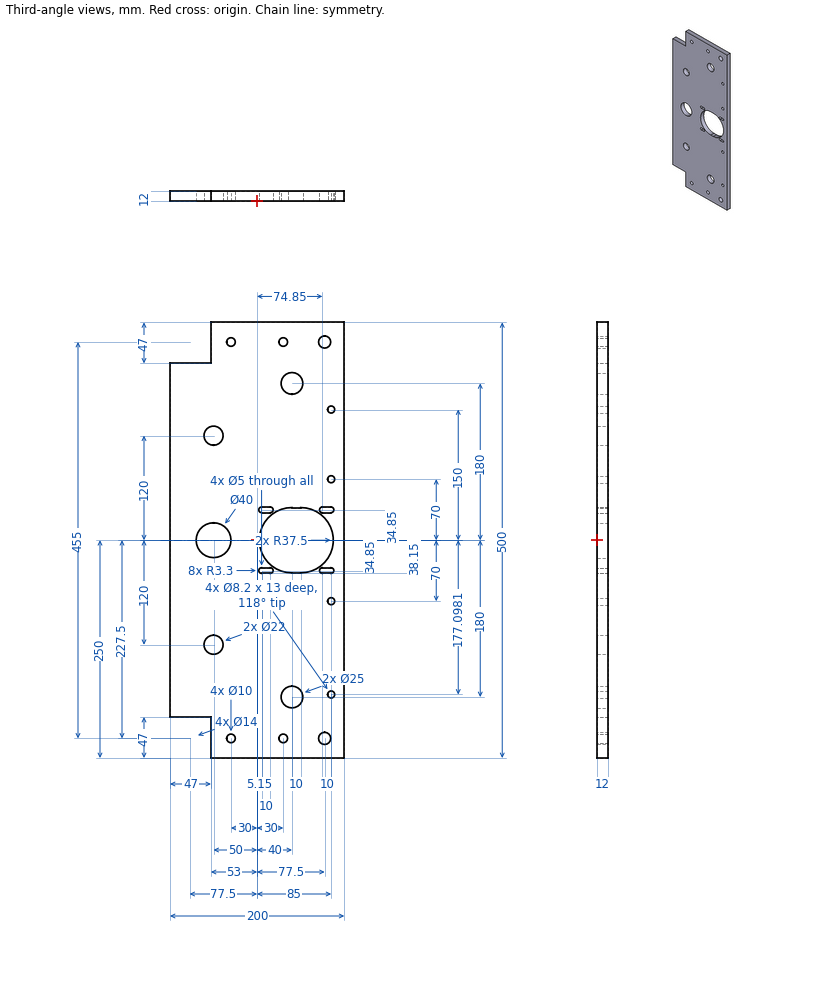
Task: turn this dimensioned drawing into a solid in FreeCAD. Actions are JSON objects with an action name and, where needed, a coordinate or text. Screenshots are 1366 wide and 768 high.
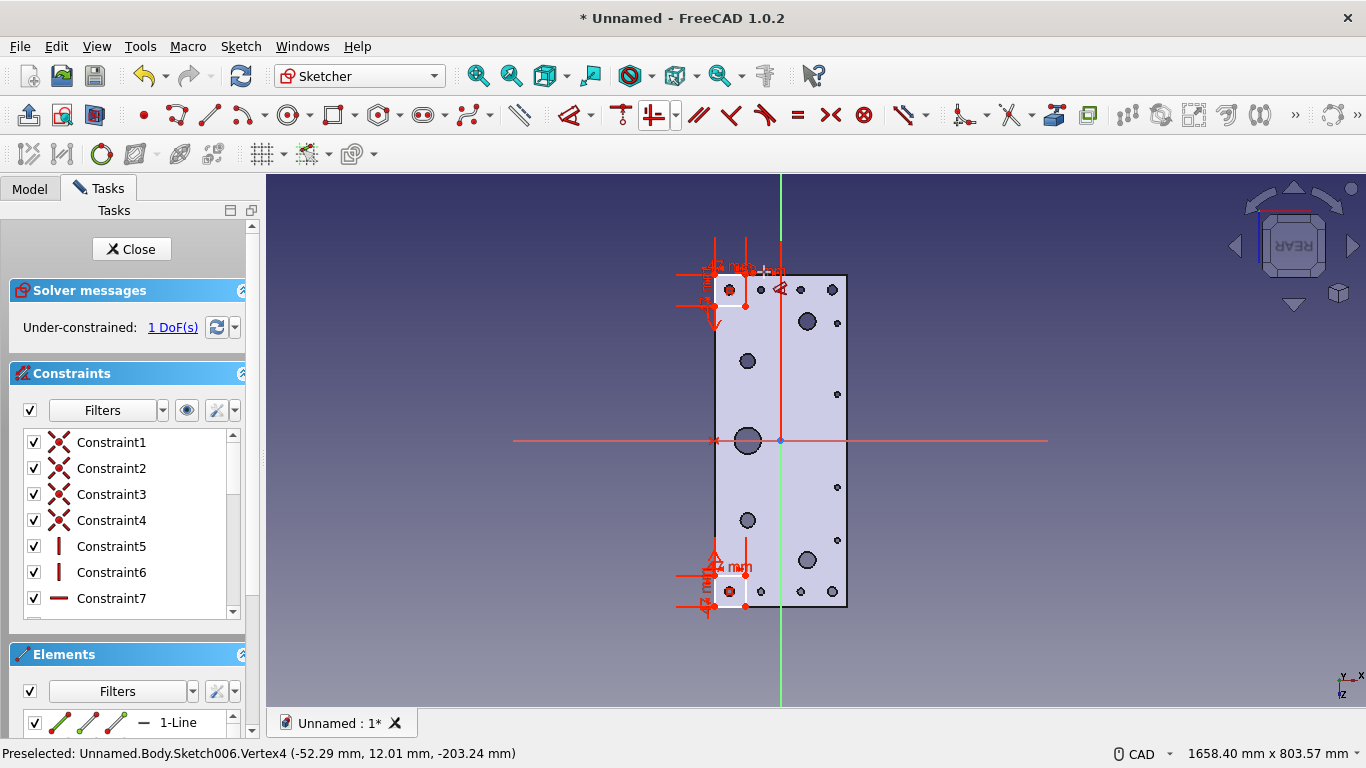
{"action": "left_click", "coordinate": [715, 275]}
{"action": "left_click", "coordinate": [815, 358]}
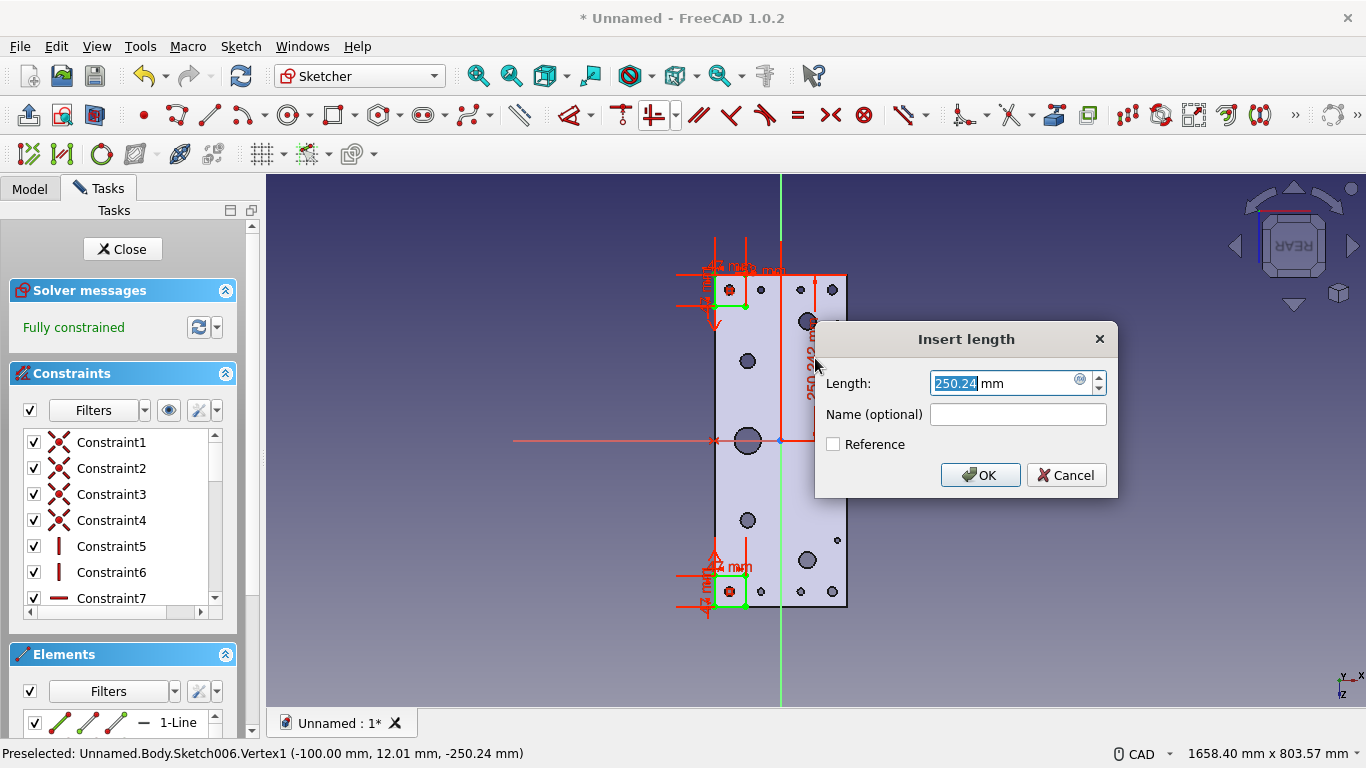
{"action": "type", "text": "250"}
{"action": "key", "text": "Return"}
{"action": "key", "text": "Escape"}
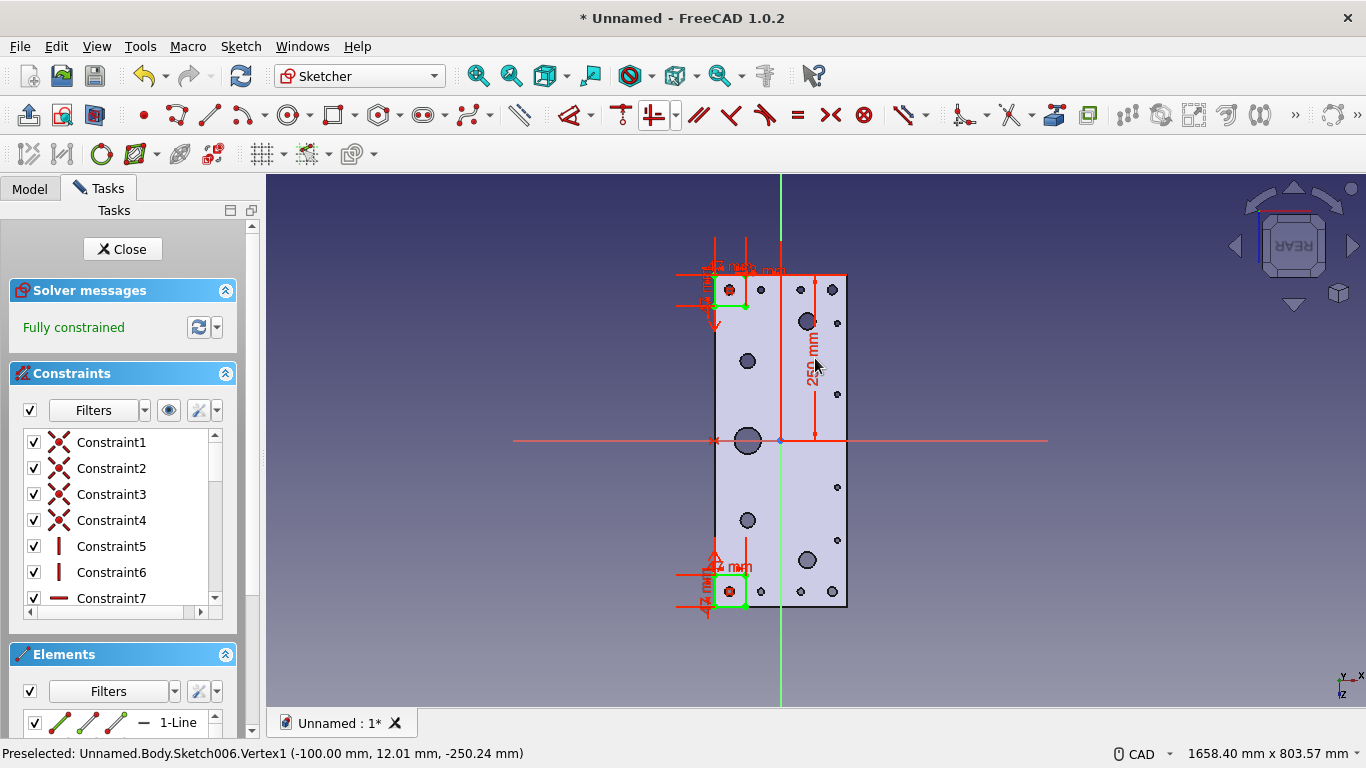
{"action": "left_click", "coordinate": [123, 249]}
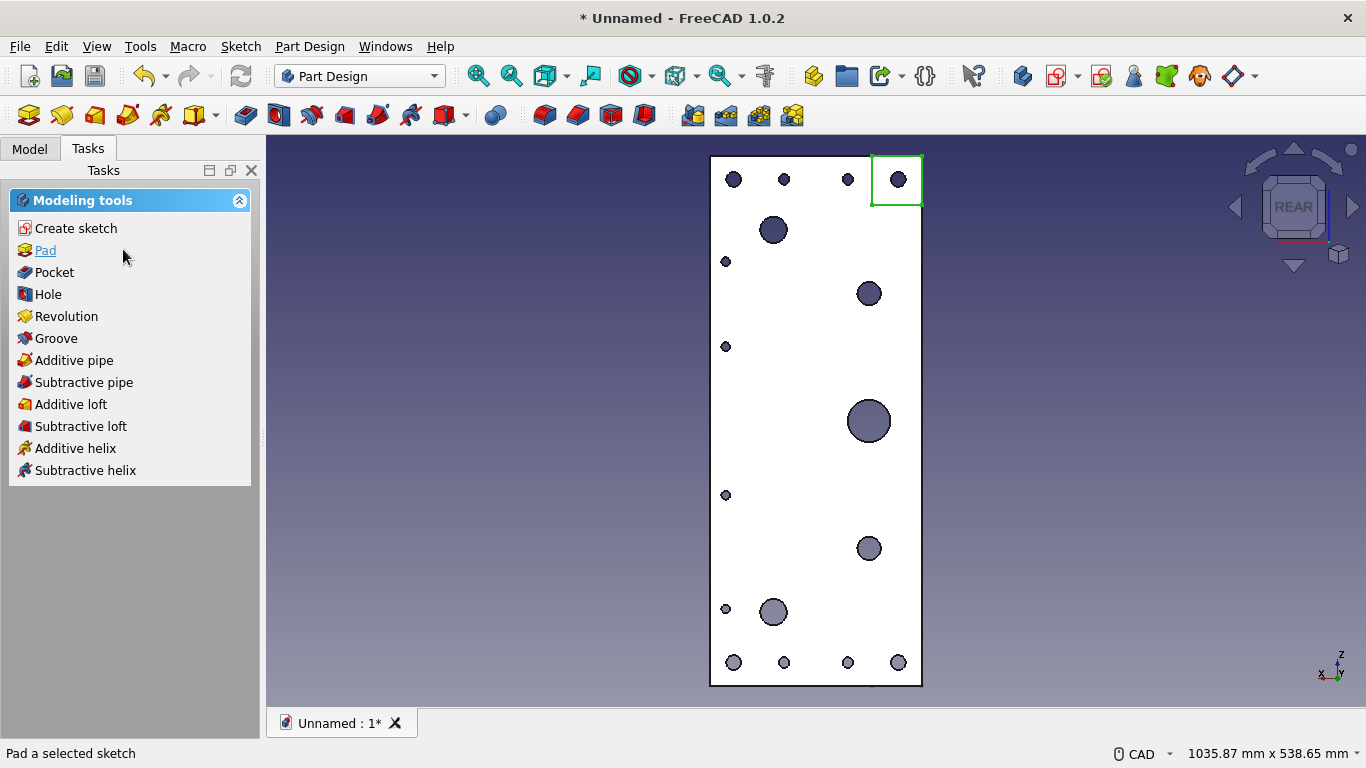
{"action": "left_click", "coordinate": [246, 116]}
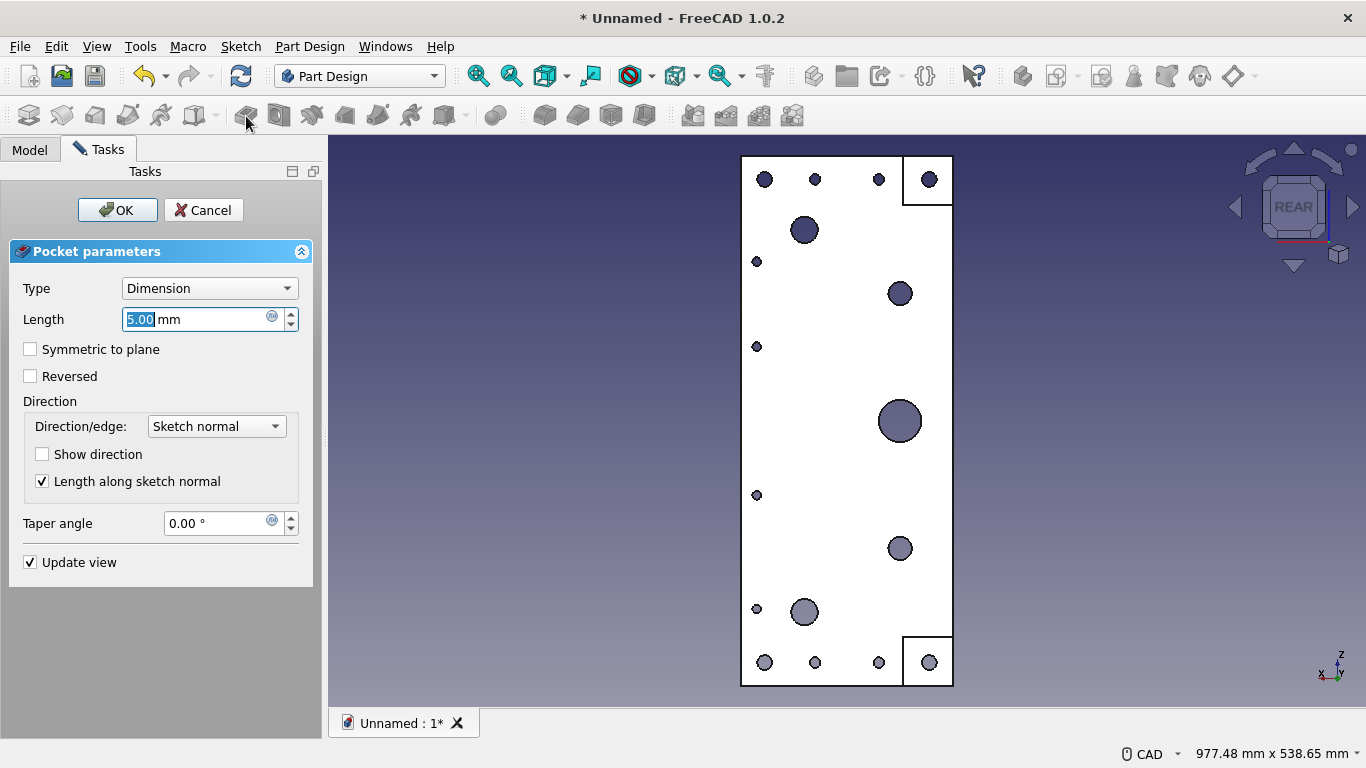
{"action": "left_click", "coordinate": [210, 288]}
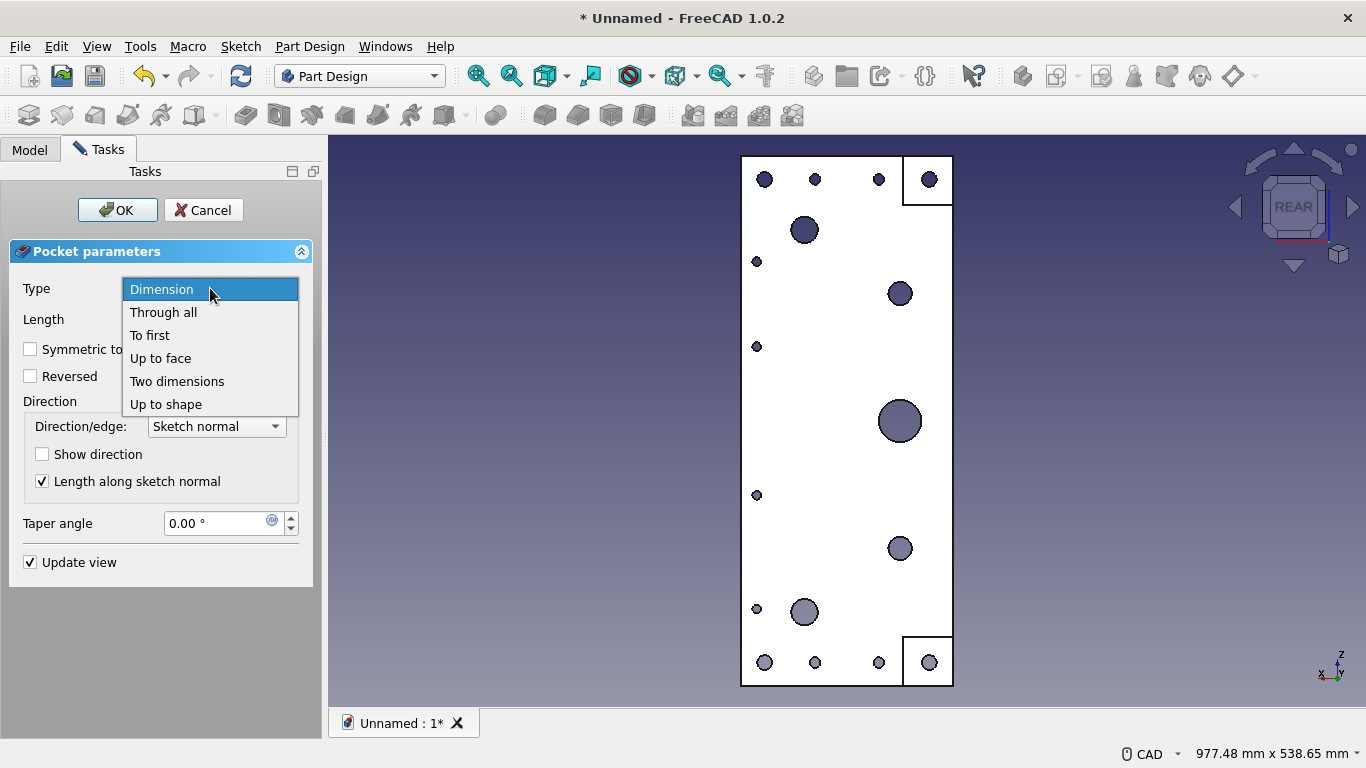
{"action": "left_click", "coordinate": [208, 312]}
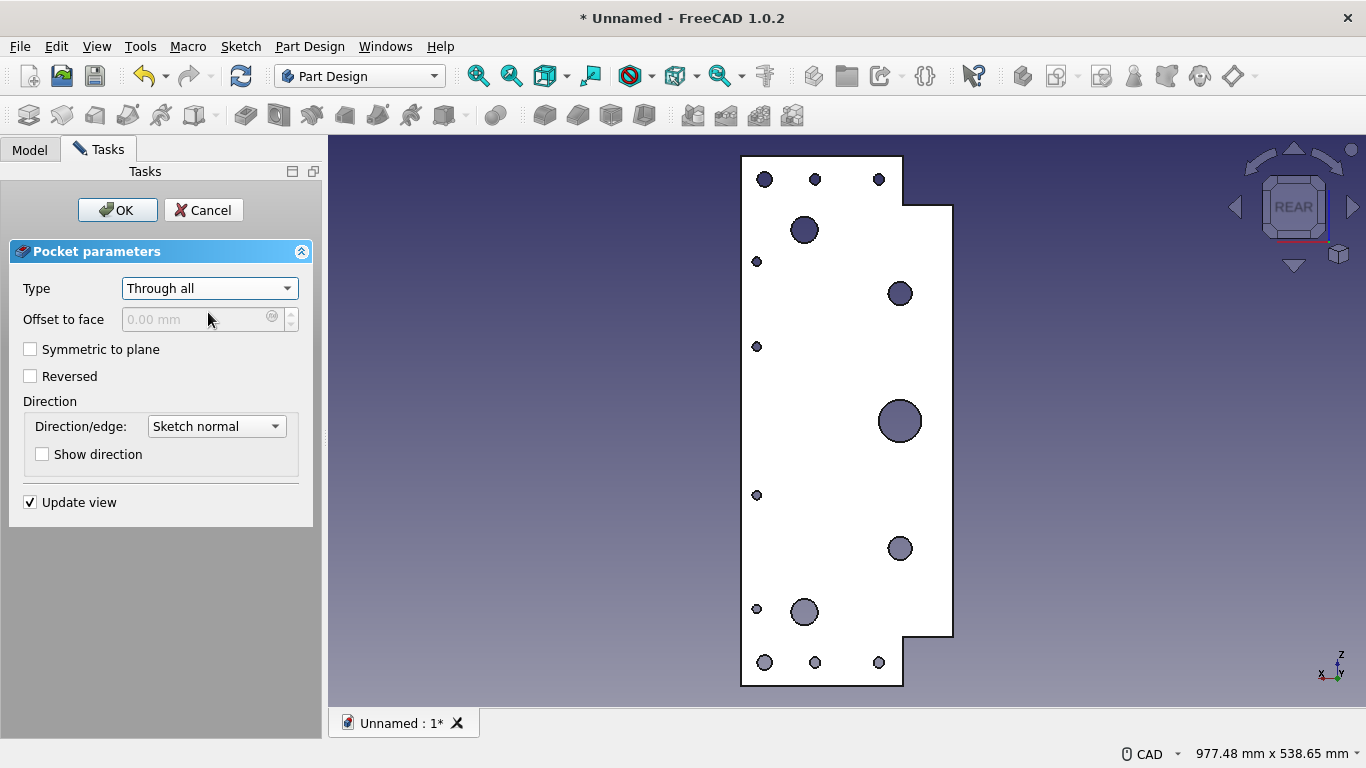
{"action": "left_click", "coordinate": [118, 210]}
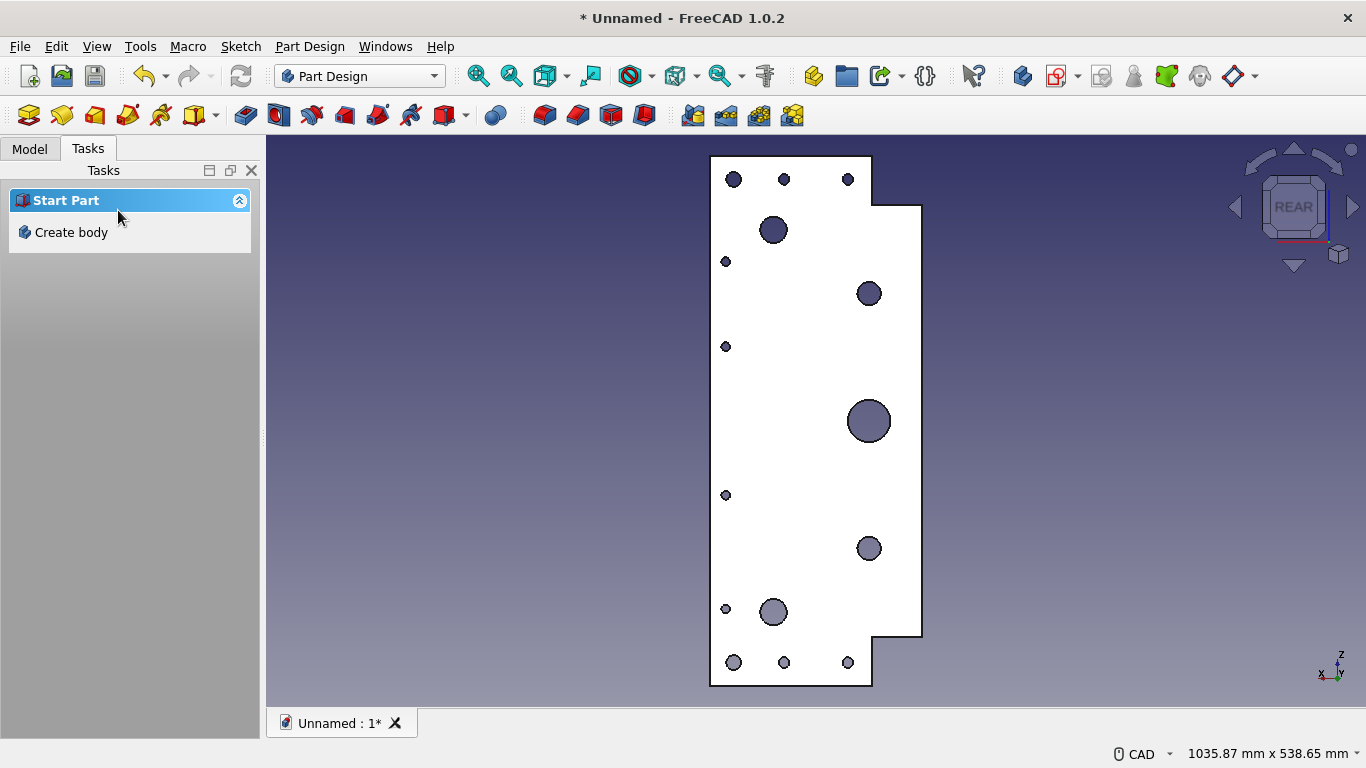
{"action": "left_click", "coordinate": [816, 496]}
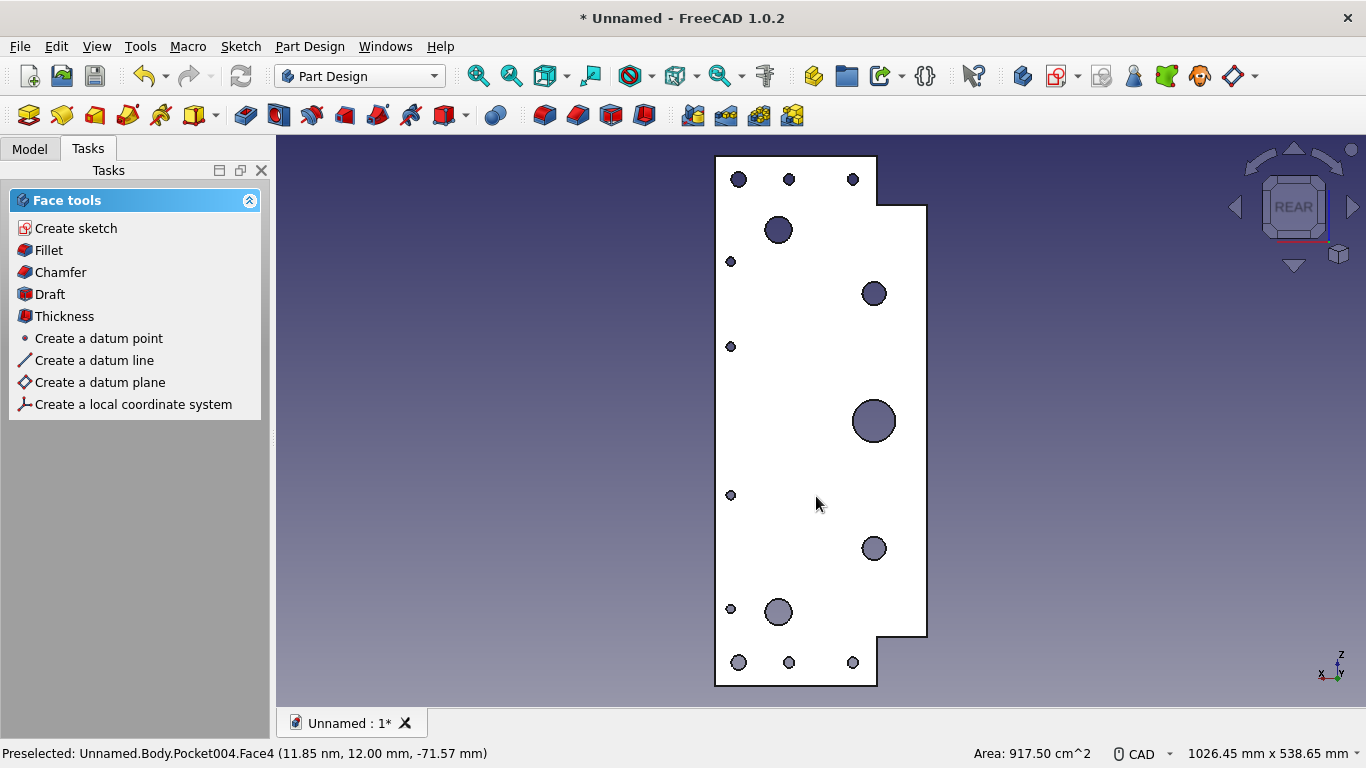
{"action": "left_click", "coordinate": [1056, 76]}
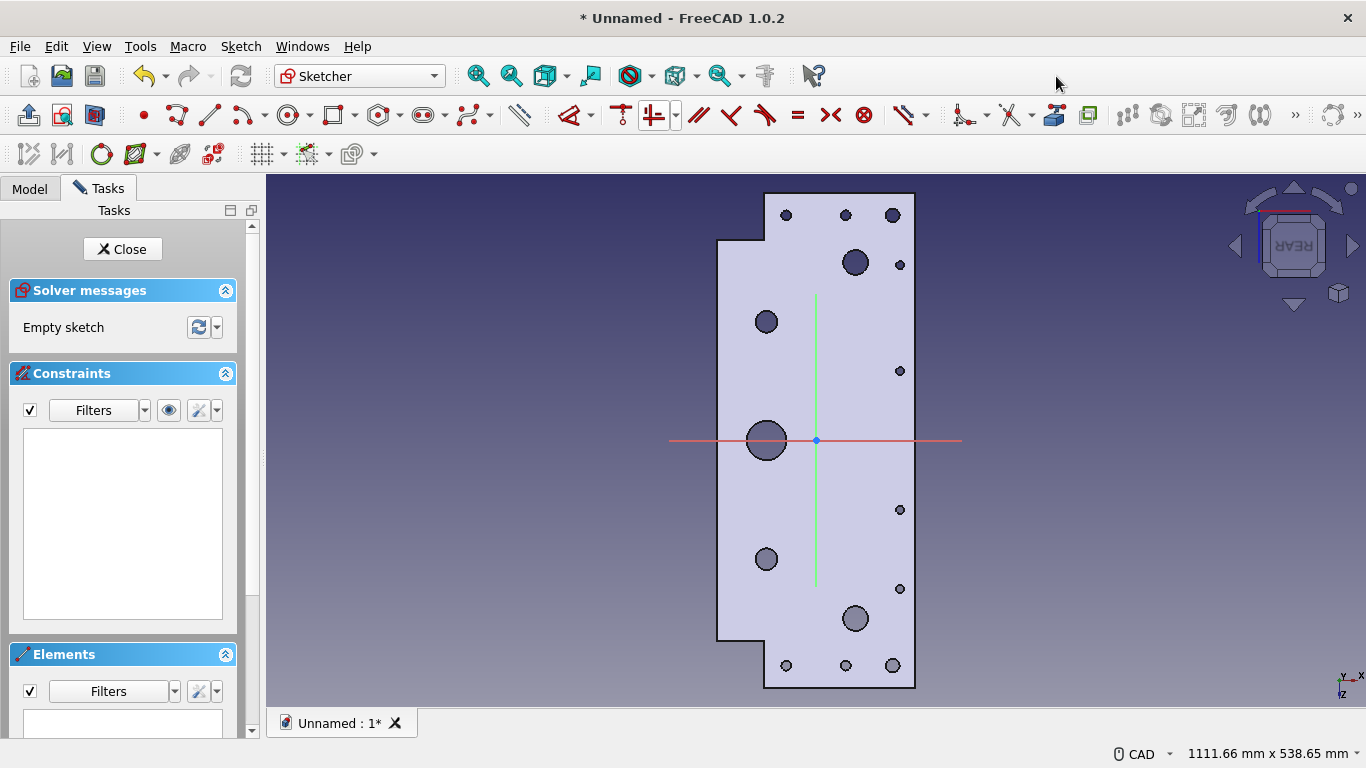
{"action": "scroll", "coordinate": [888, 440], "scroll_direction": "up", "scroll_amount": 8}